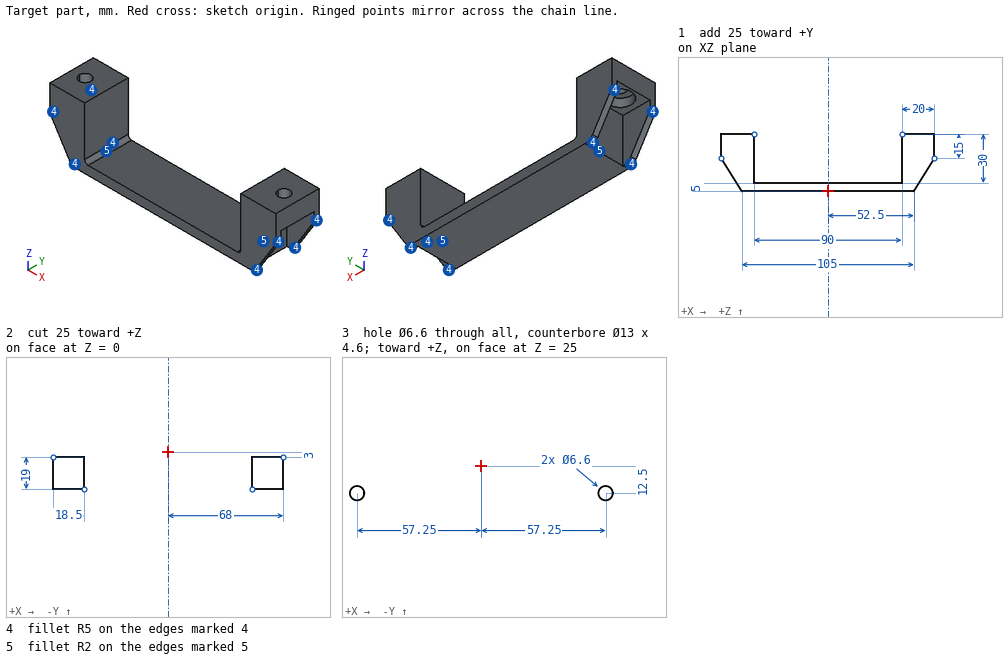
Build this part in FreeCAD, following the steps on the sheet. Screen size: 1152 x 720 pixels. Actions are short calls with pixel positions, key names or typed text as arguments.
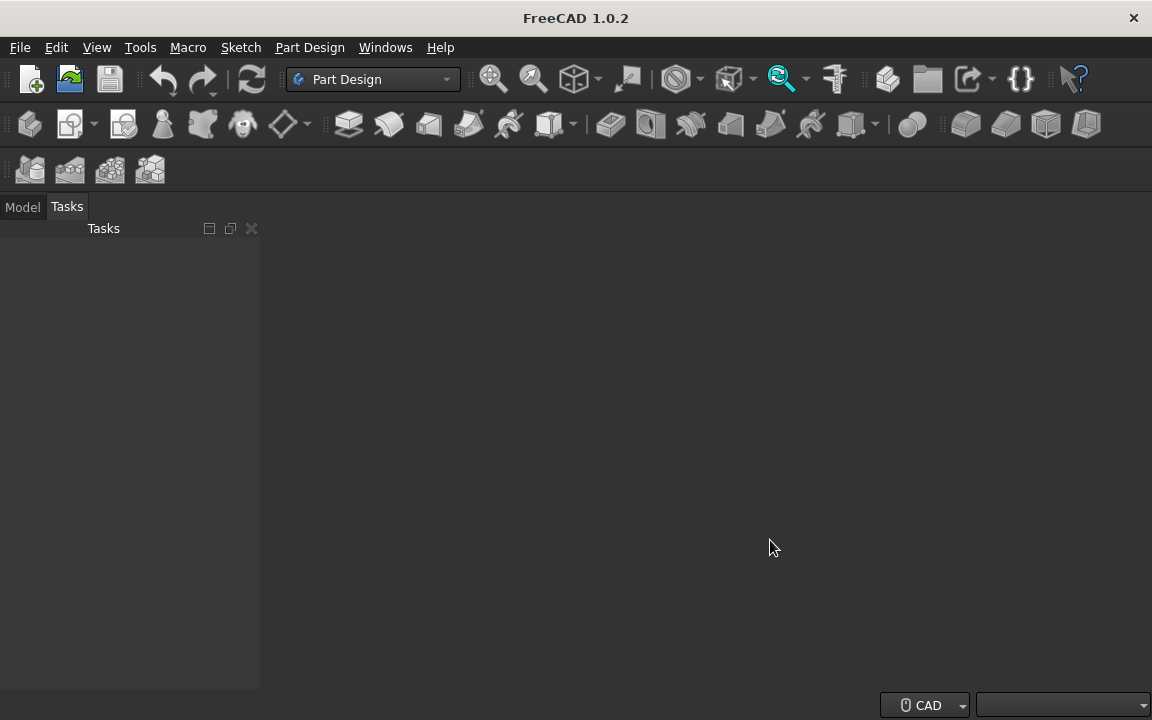
click(30, 80)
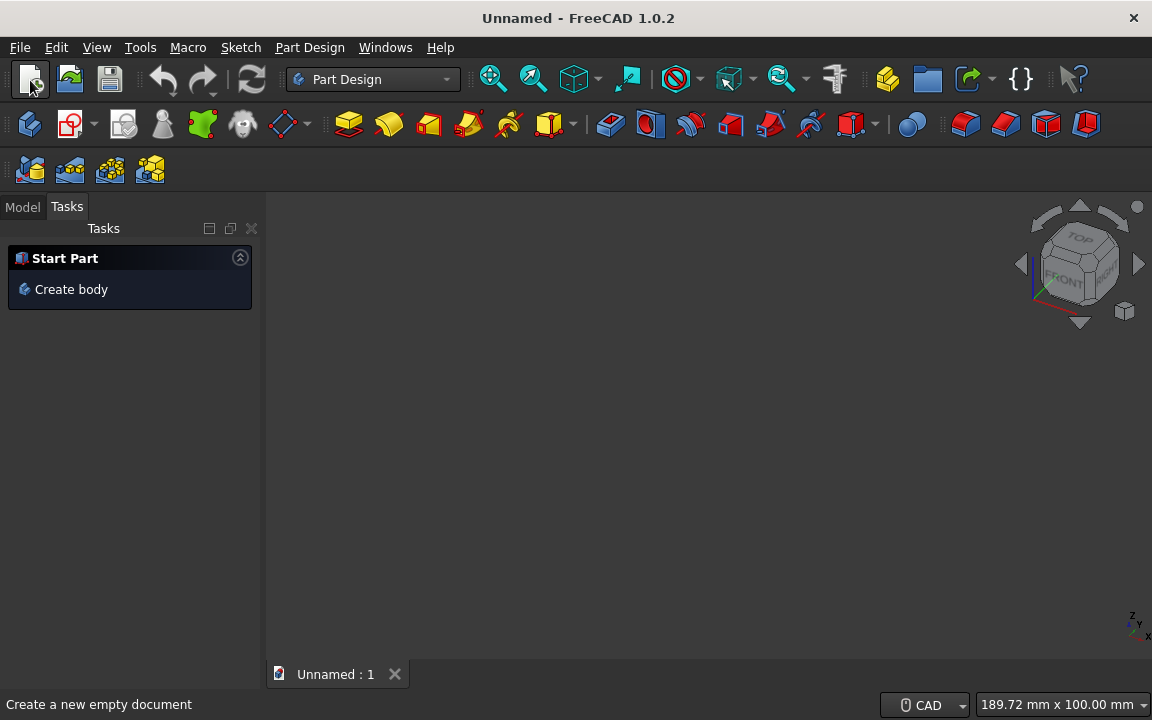
click(70, 124)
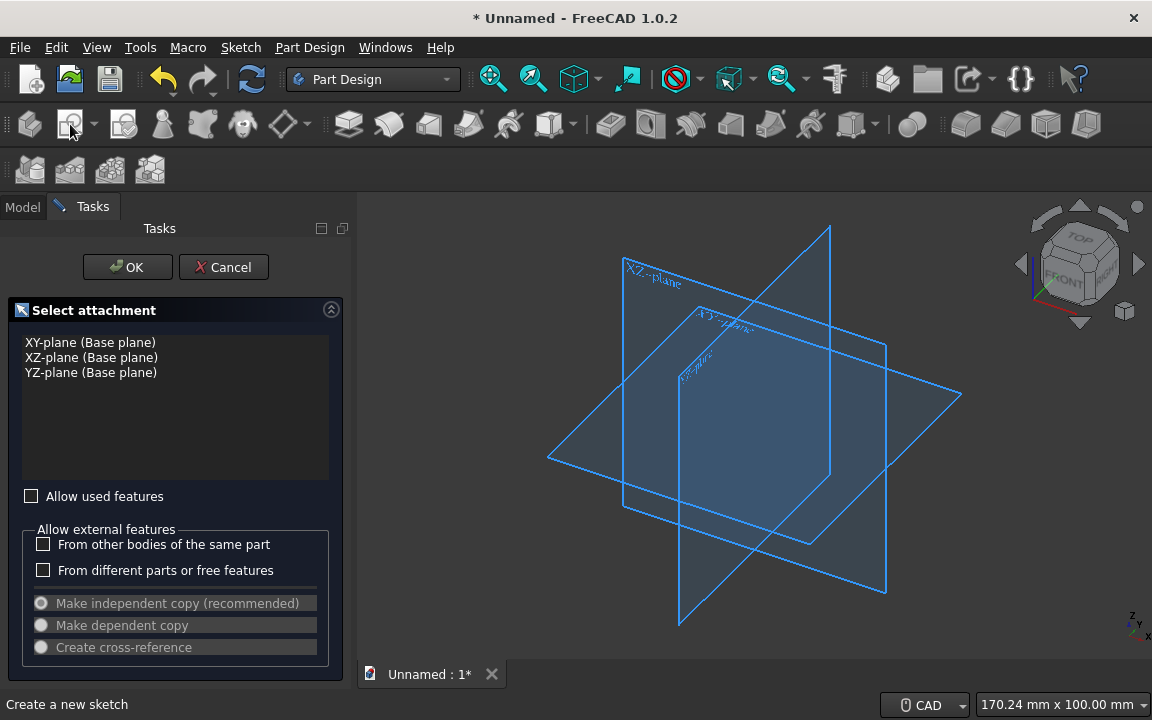
click(82, 358)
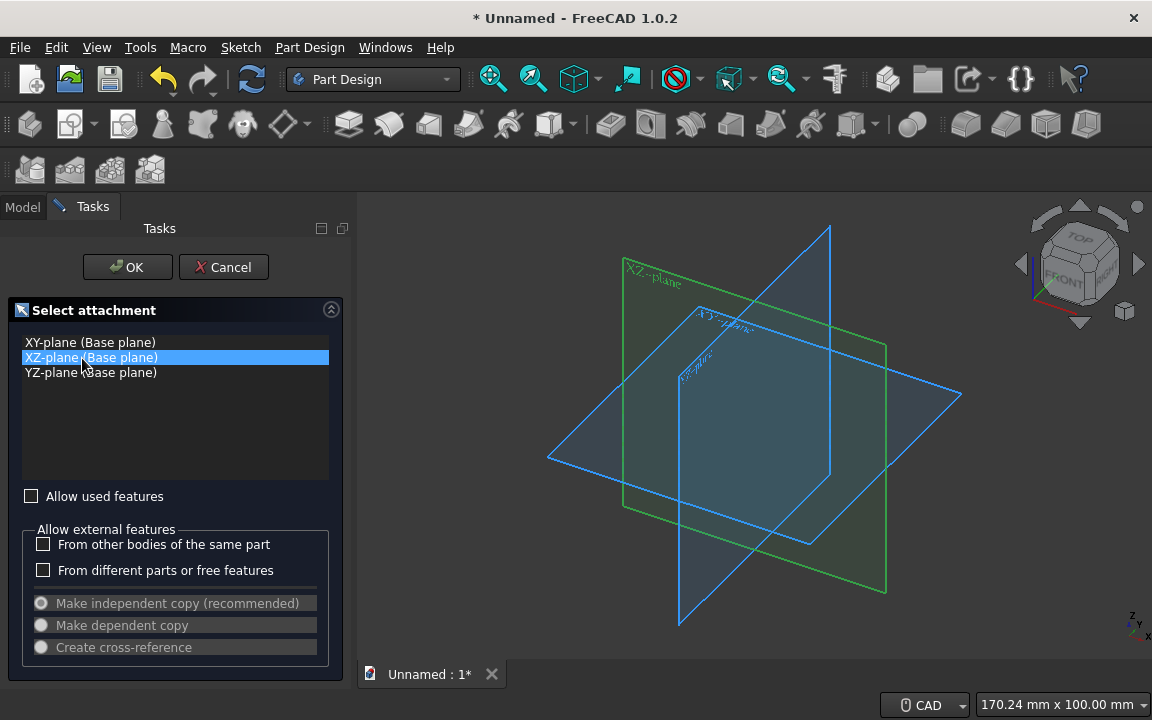
click(128, 267)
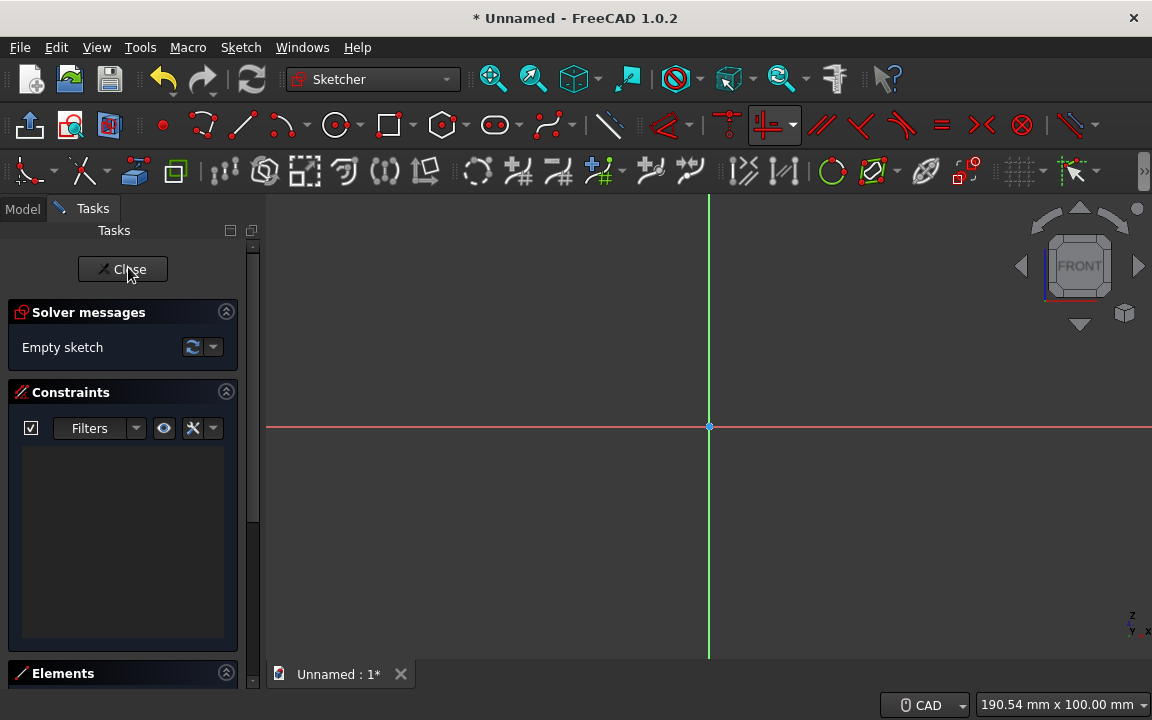
scroll(331, 631, down, 1)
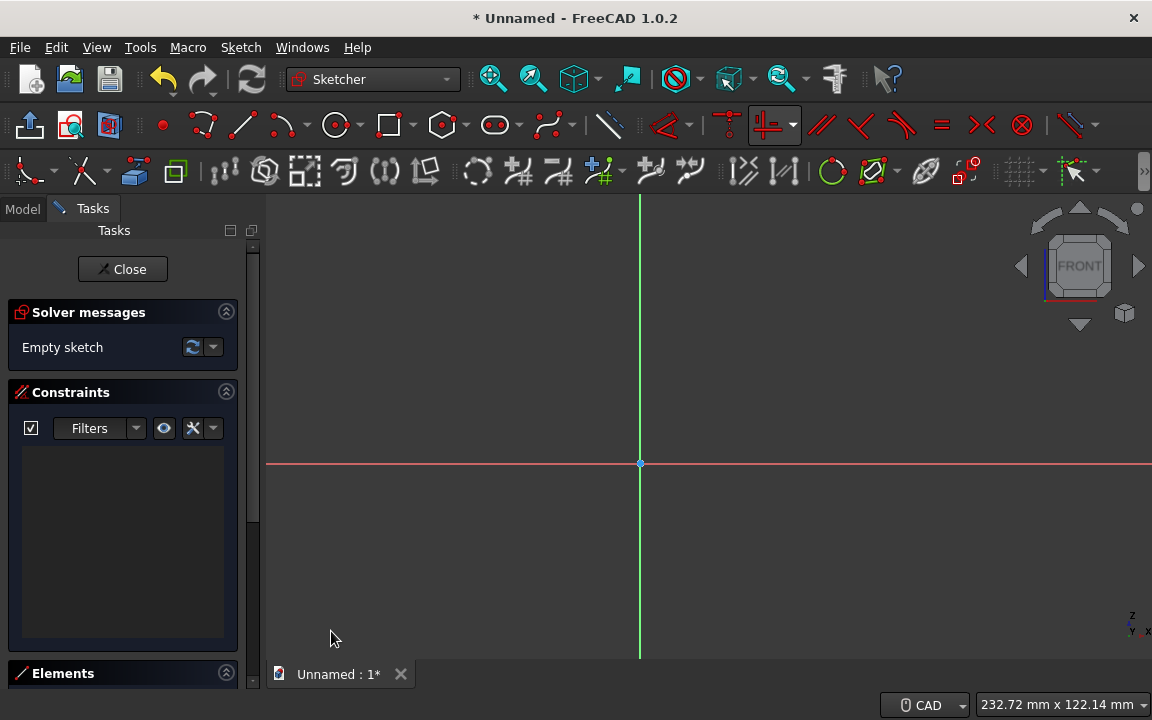
key(g)
key(m)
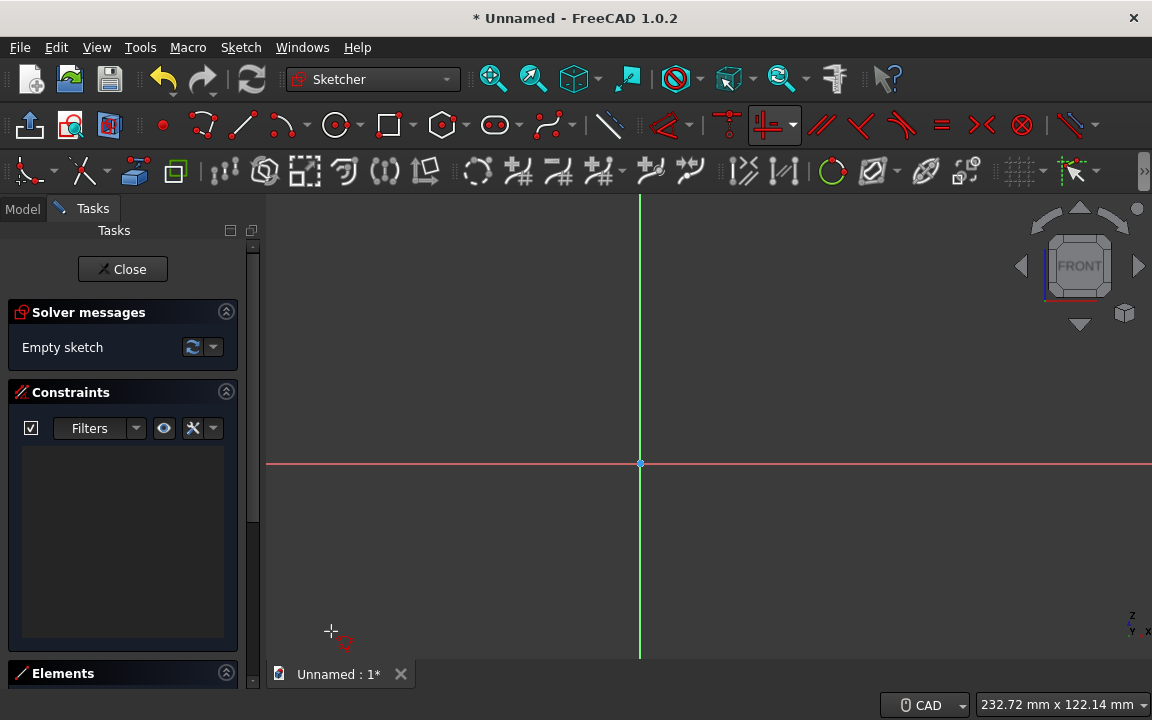
click(469, 445)
click(812, 445)
click(812, 330)
click(888, 330)
click(888, 388)
click(840, 464)
click(441, 455)
click(393, 388)
click(393, 330)
click(469, 330)
click(469, 446)
key(Escape)
key(Escape)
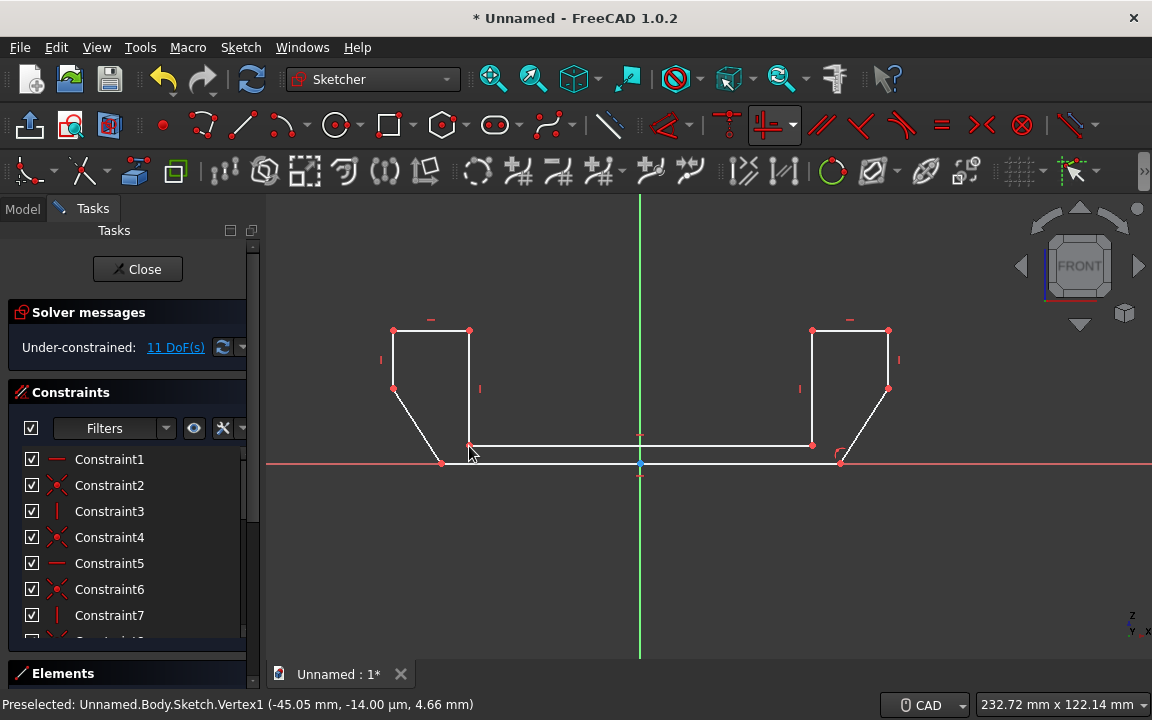
click(888, 389)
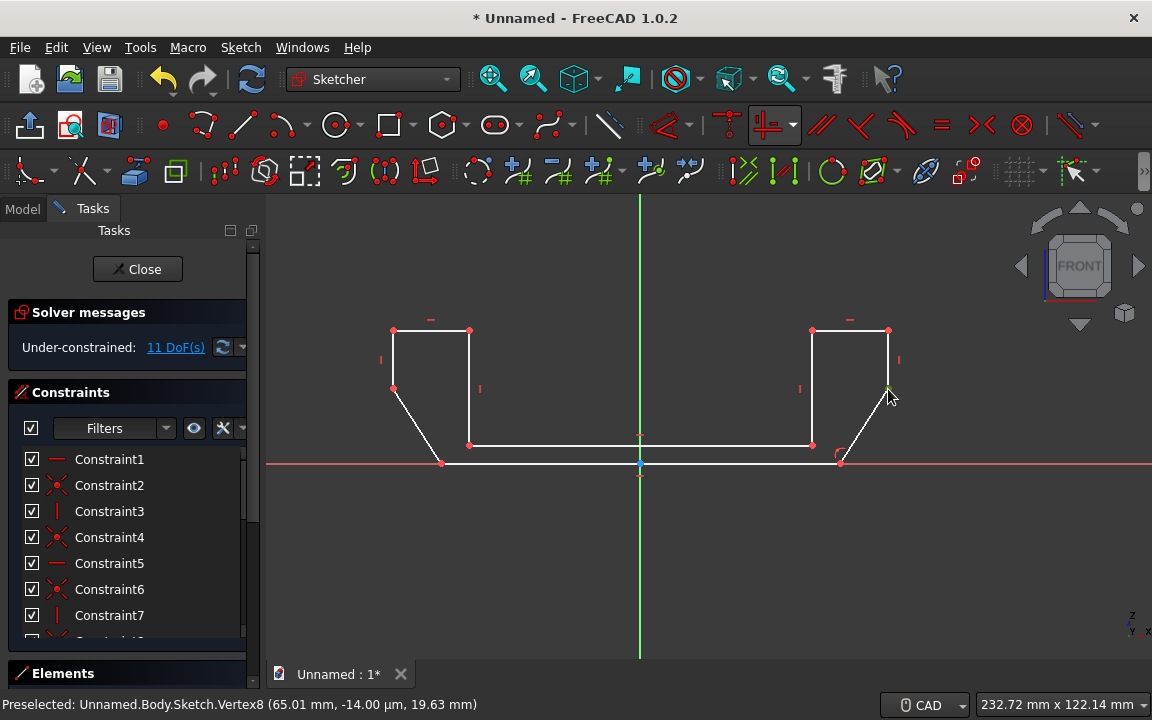
click(393, 389)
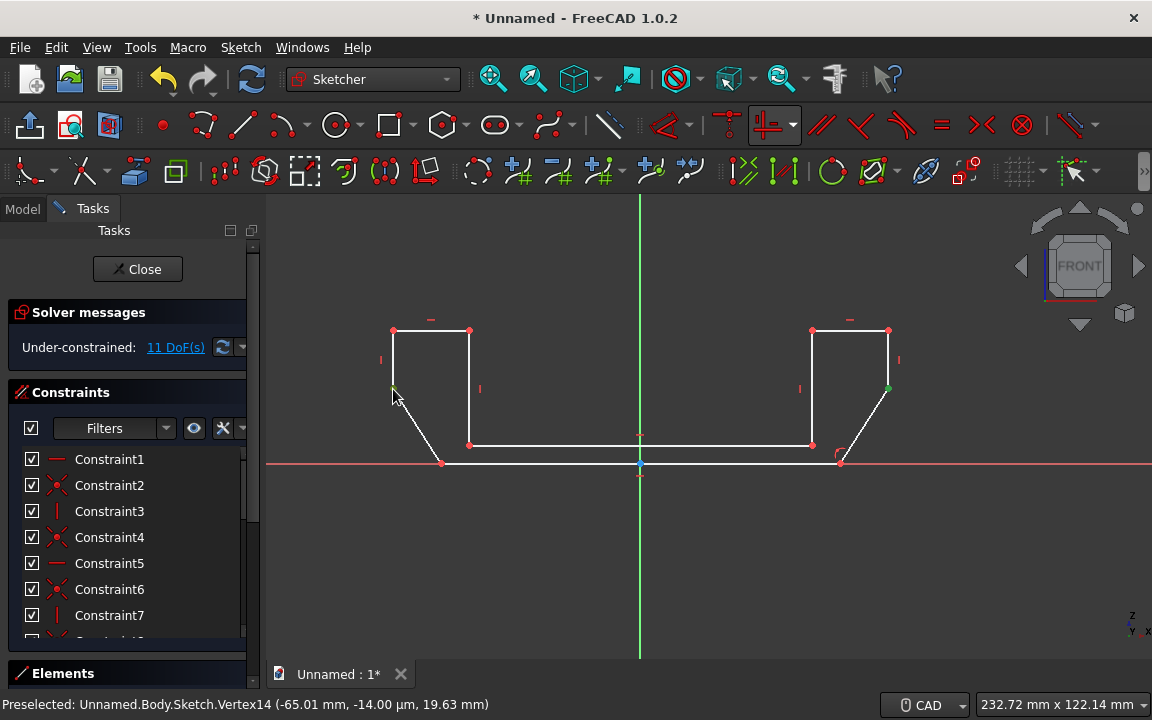
click(640, 602)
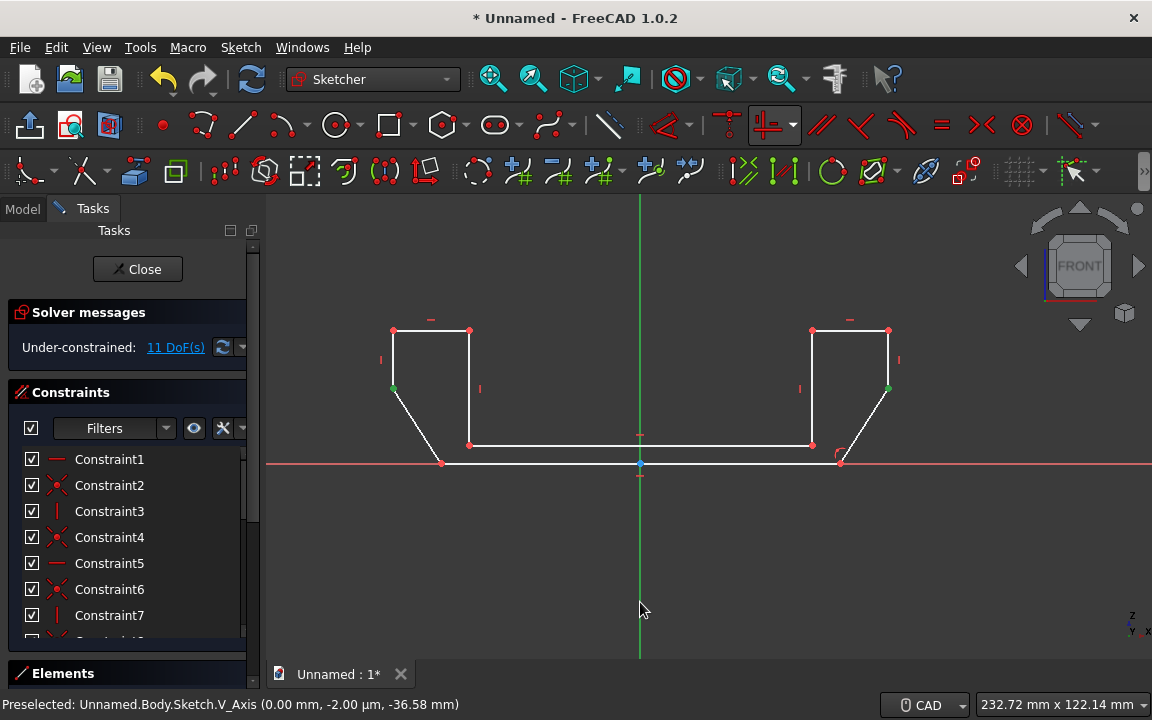
click(982, 126)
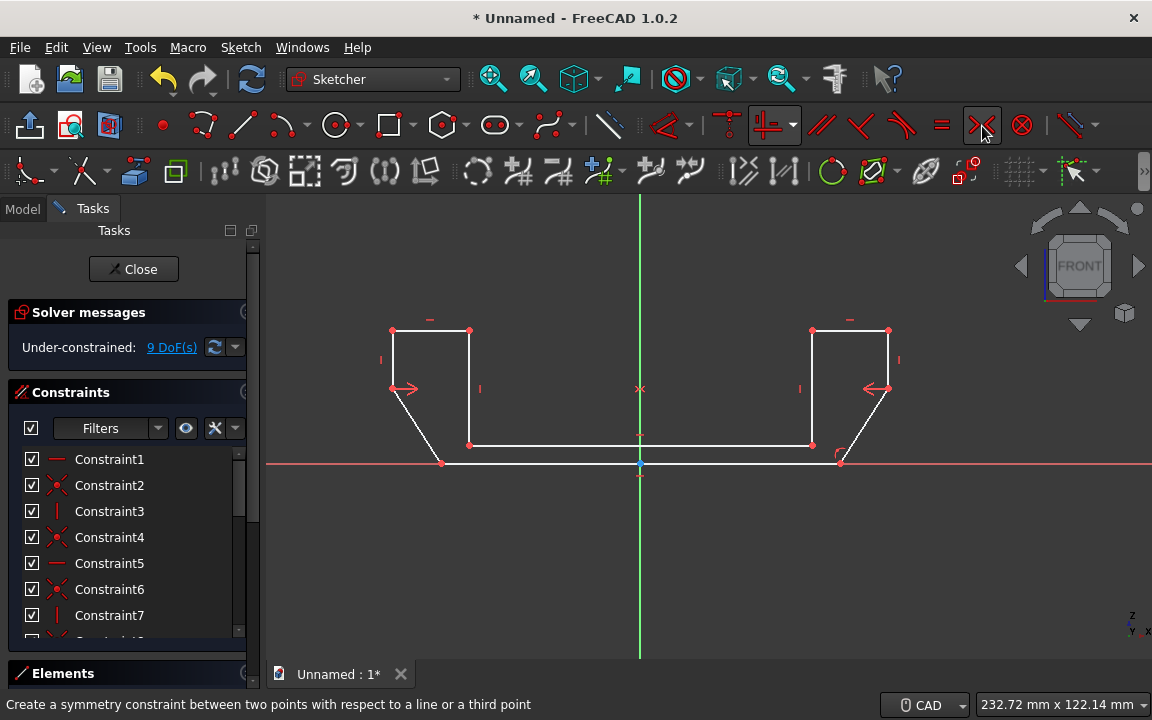
click(812, 331)